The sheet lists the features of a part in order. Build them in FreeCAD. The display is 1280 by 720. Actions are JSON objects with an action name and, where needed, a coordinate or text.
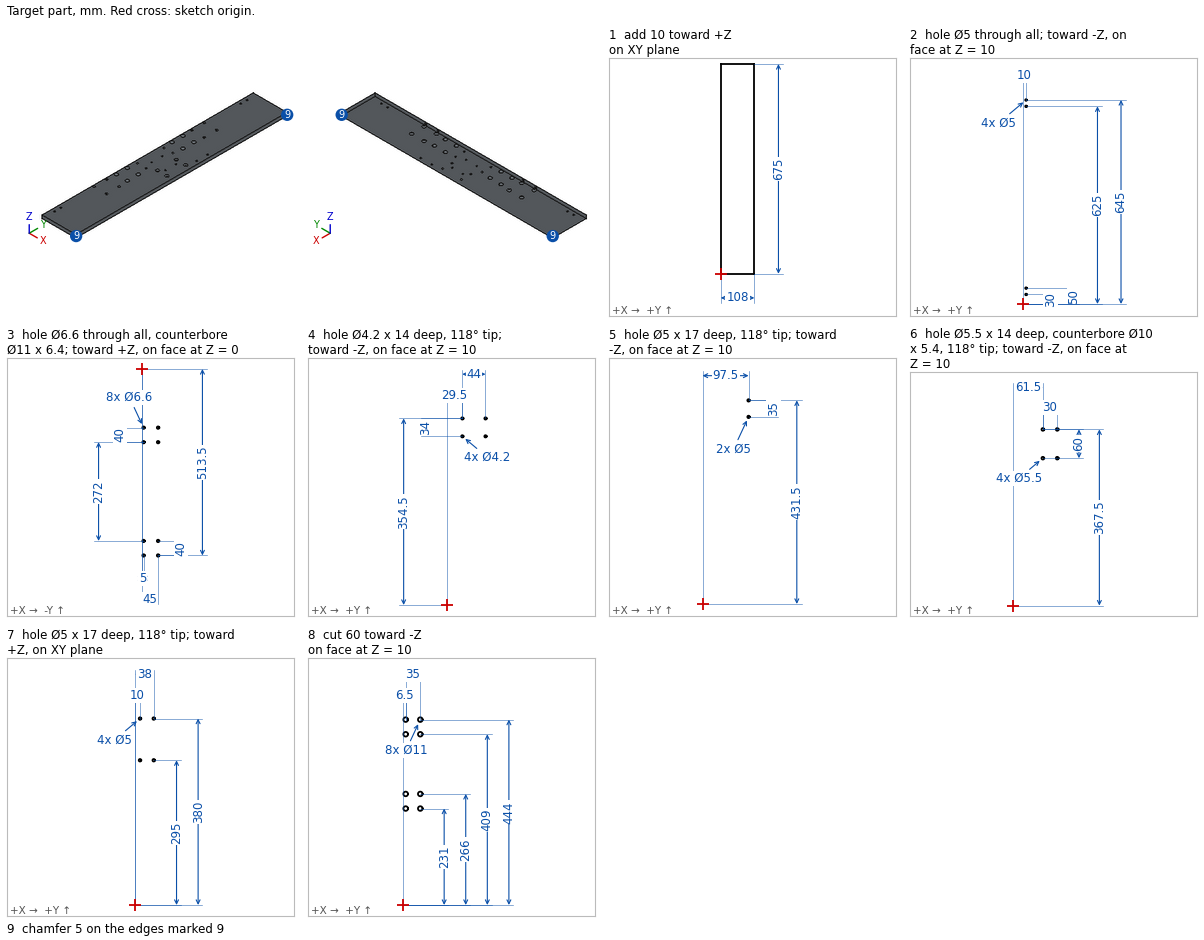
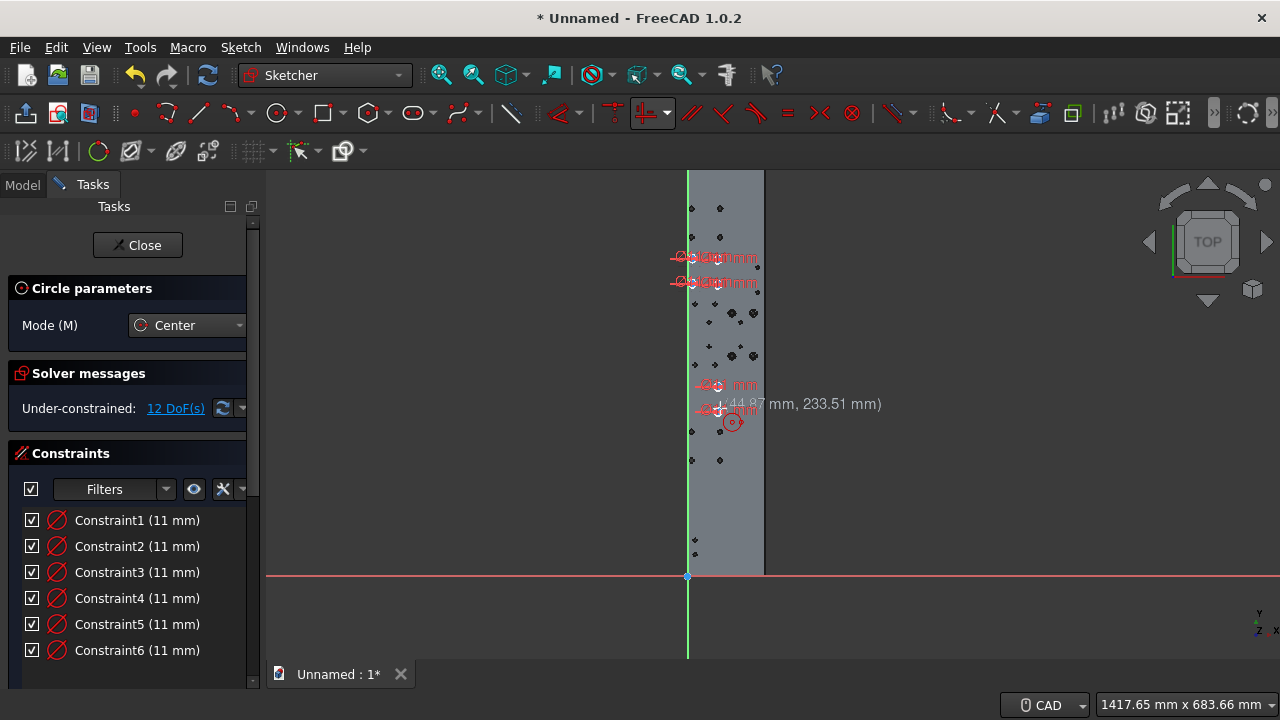
{"action": "scroll", "coordinate": [693, 411], "scroll_direction": "up", "scroll_amount": 9}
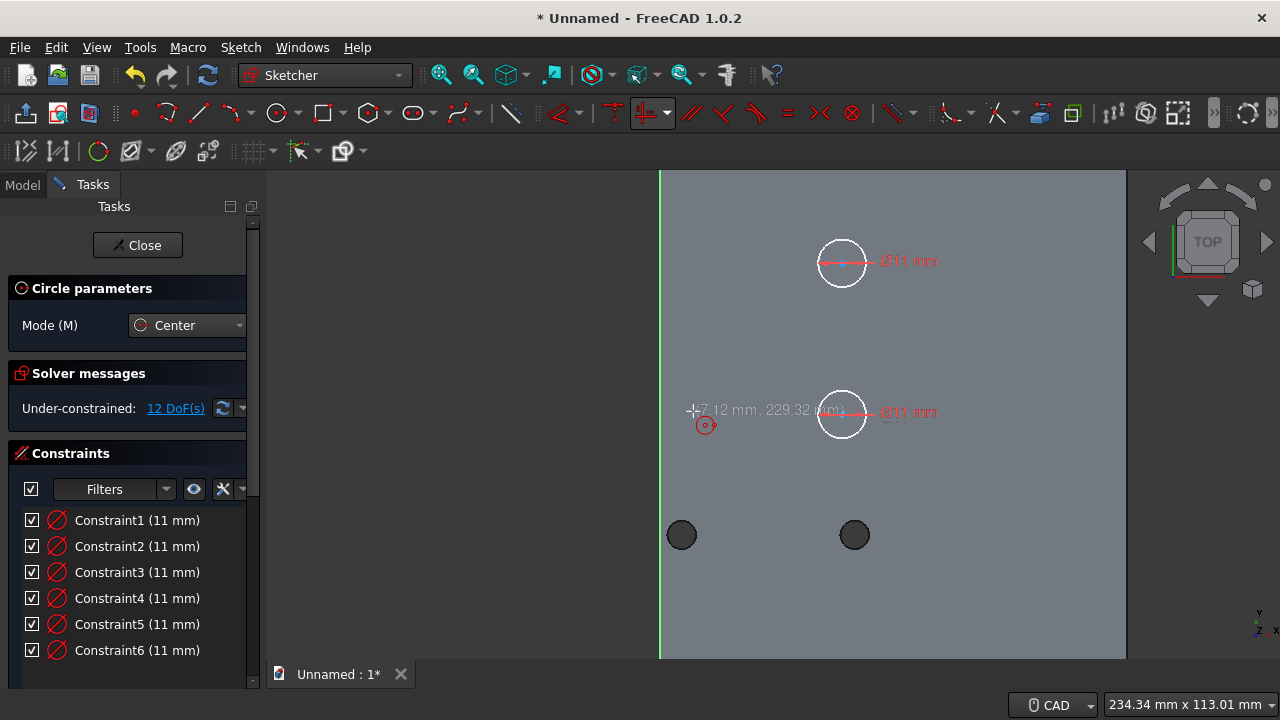
{"action": "left_click", "coordinate": [688, 407]}
{"action": "mouse_move", "coordinate": [705, 390]}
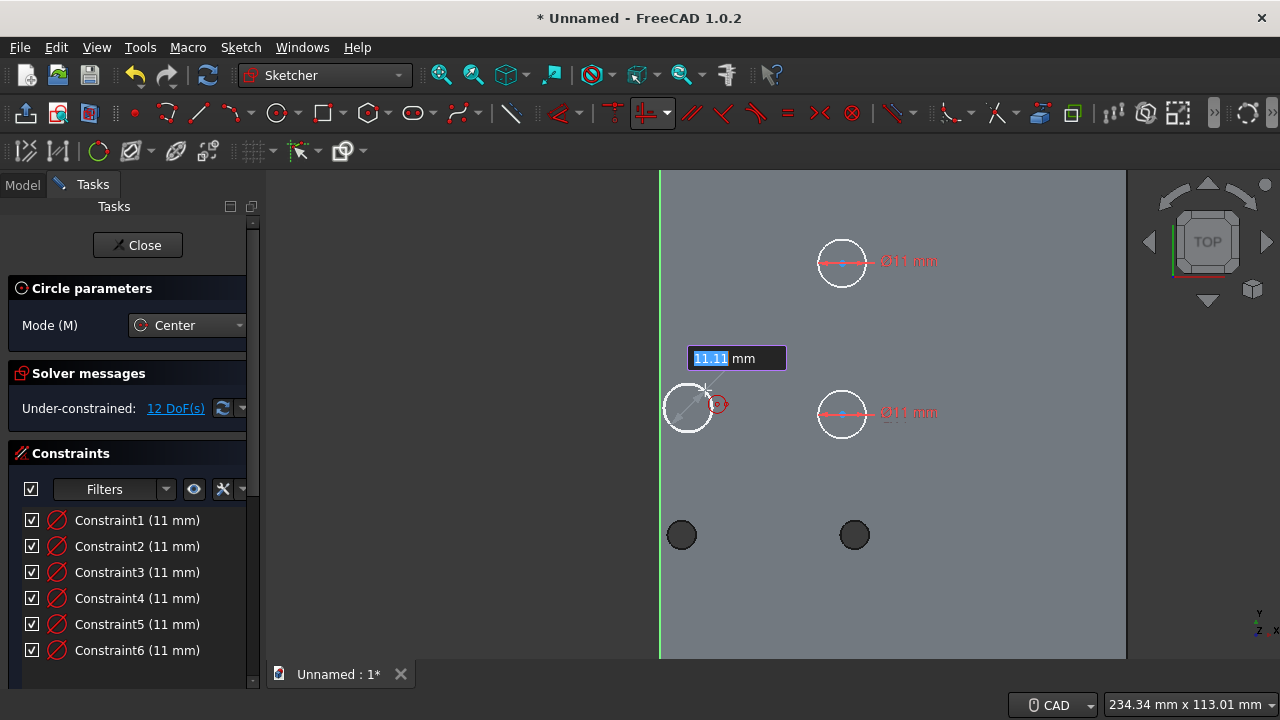
{"action": "type", "text": "11"}
{"action": "key", "text": "Return"}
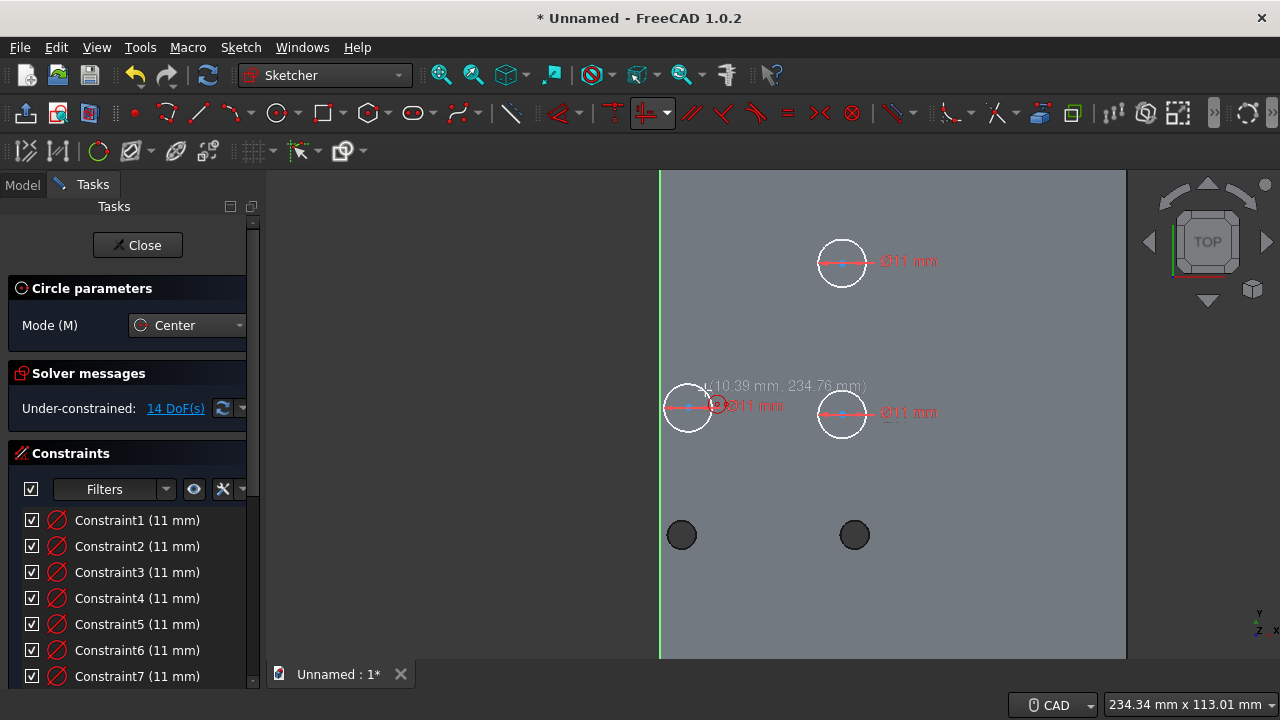
{"action": "left_click", "coordinate": [688, 256]}
{"action": "mouse_move", "coordinate": [705, 239]}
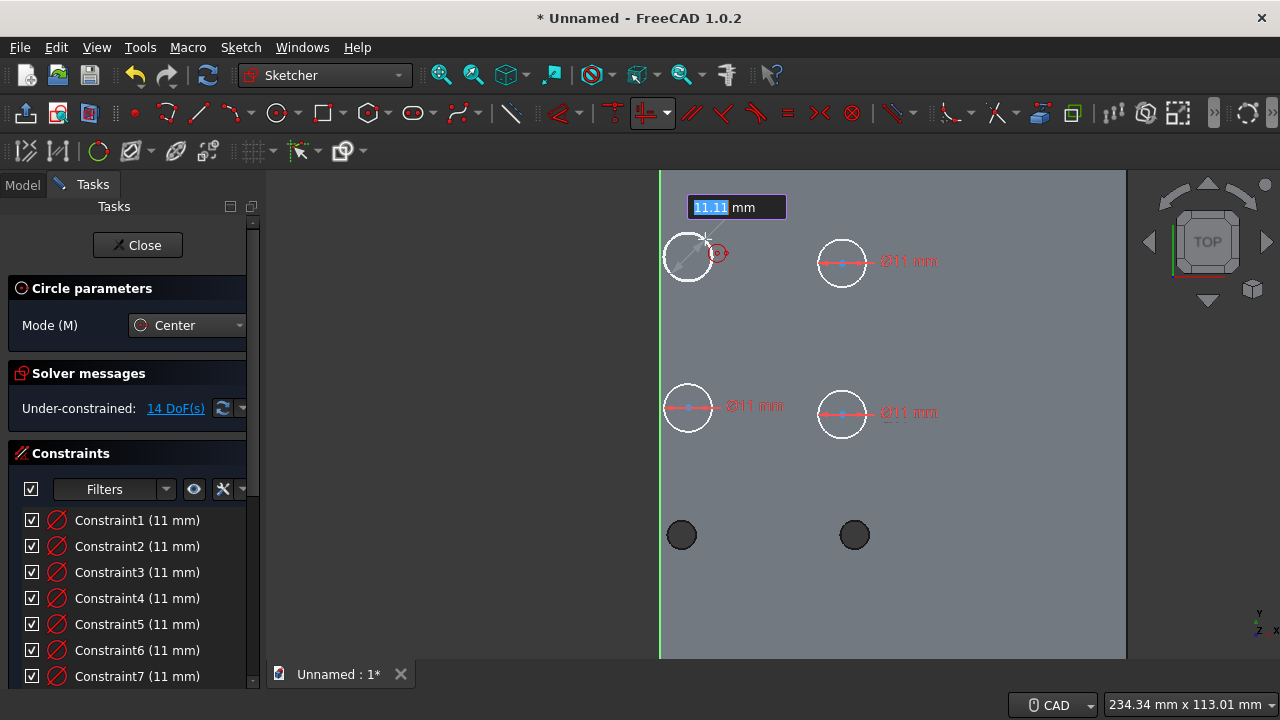
{"action": "type", "text": "11"}
{"action": "key", "text": "Return"}
{"action": "key", "text": "Escape"}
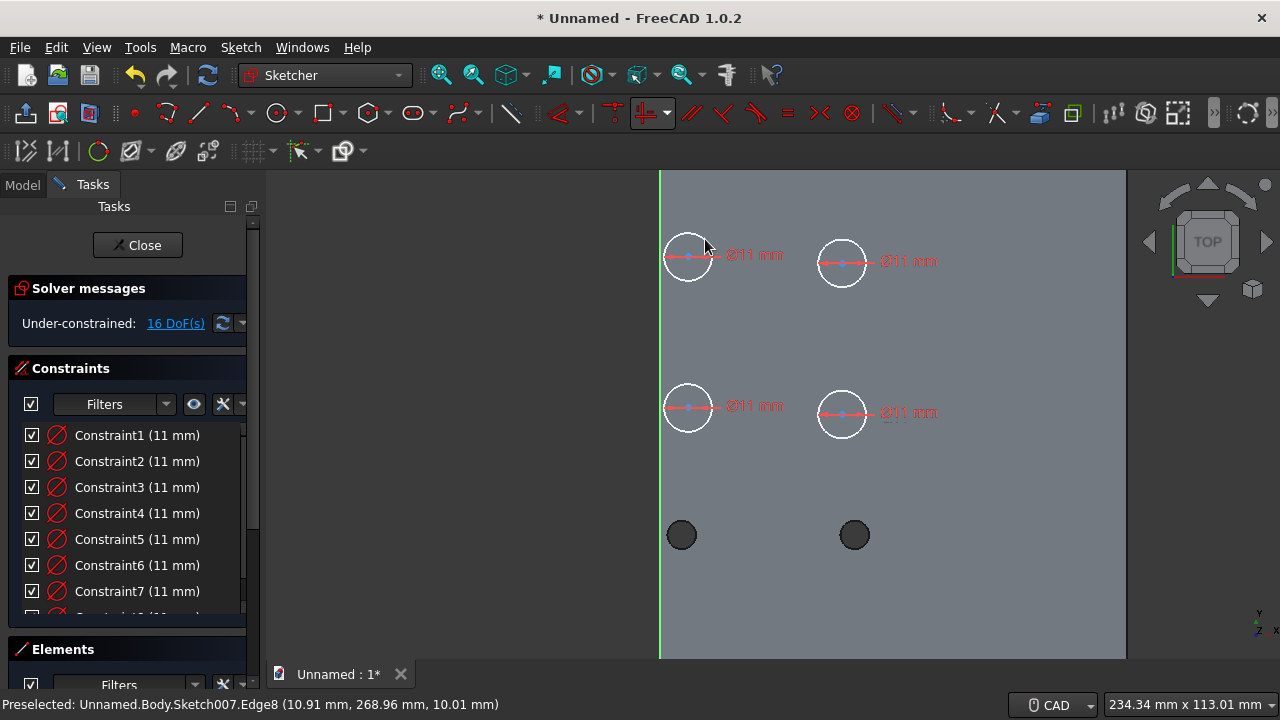
{"action": "scroll", "coordinate": [693, 411], "scroll_direction": "down", "scroll_amount": 9}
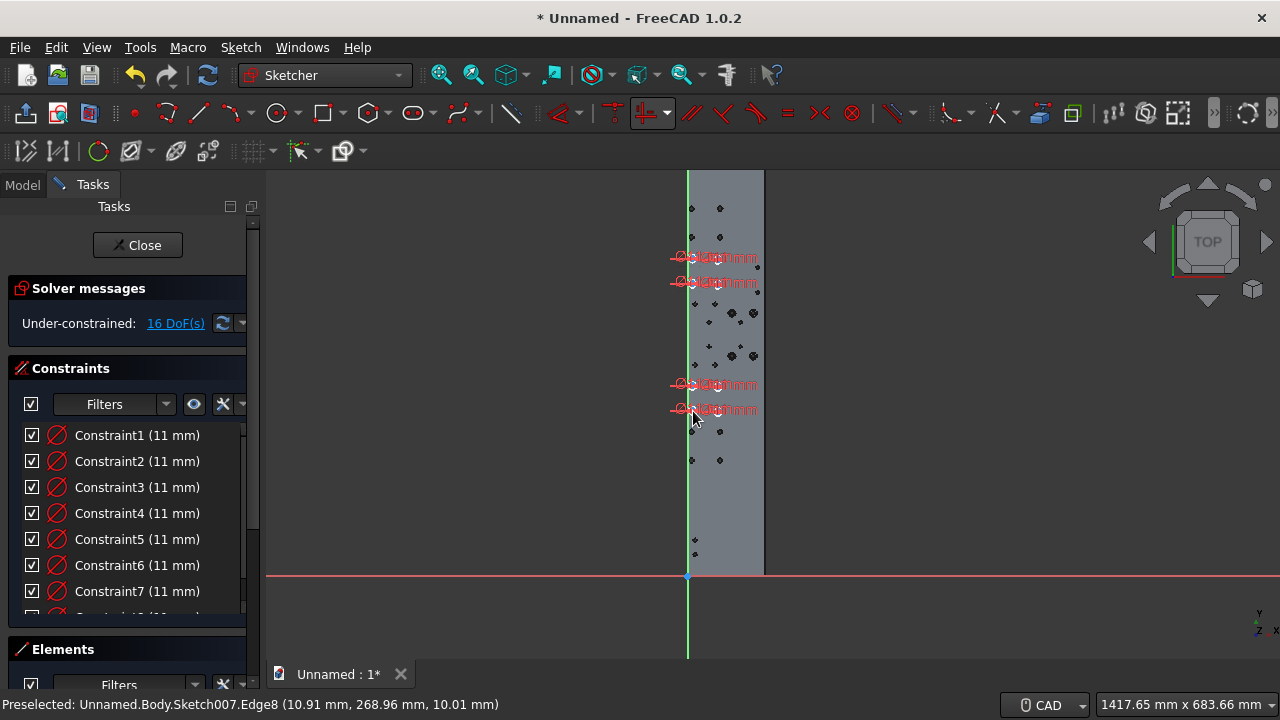
{"action": "left_click", "coordinate": [718, 260]}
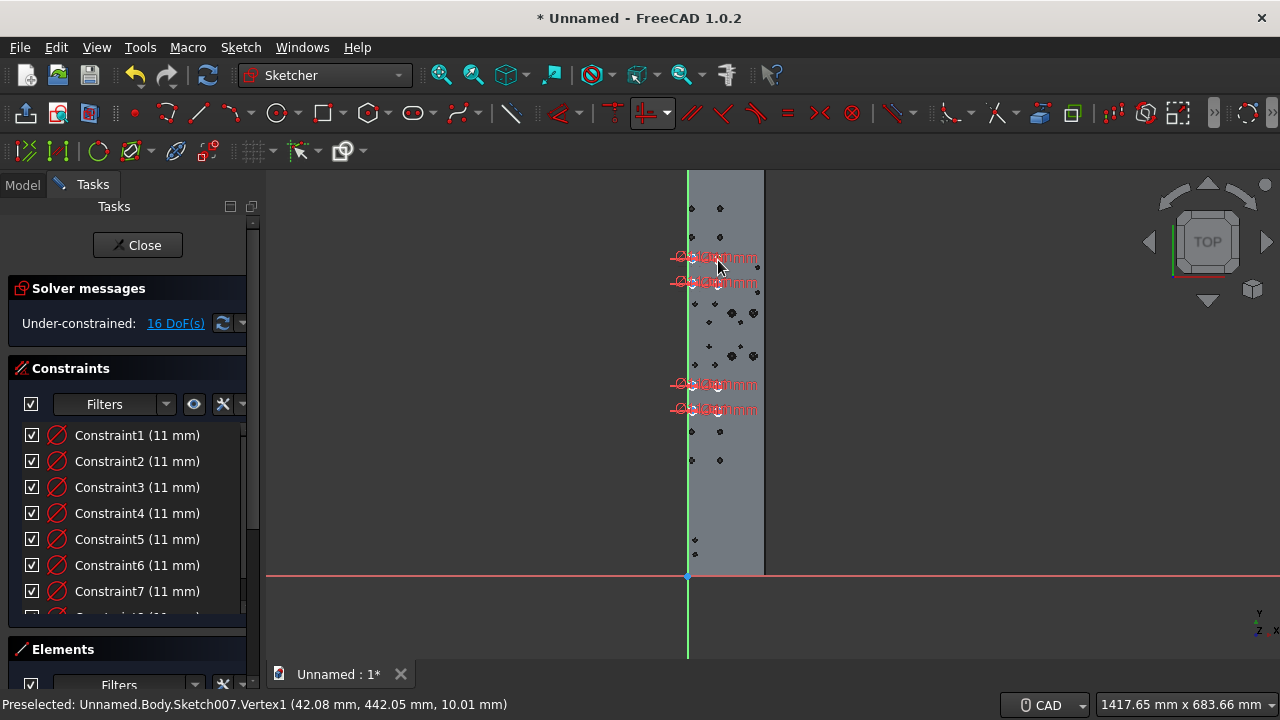
{"action": "left_click", "coordinate": [693, 259]}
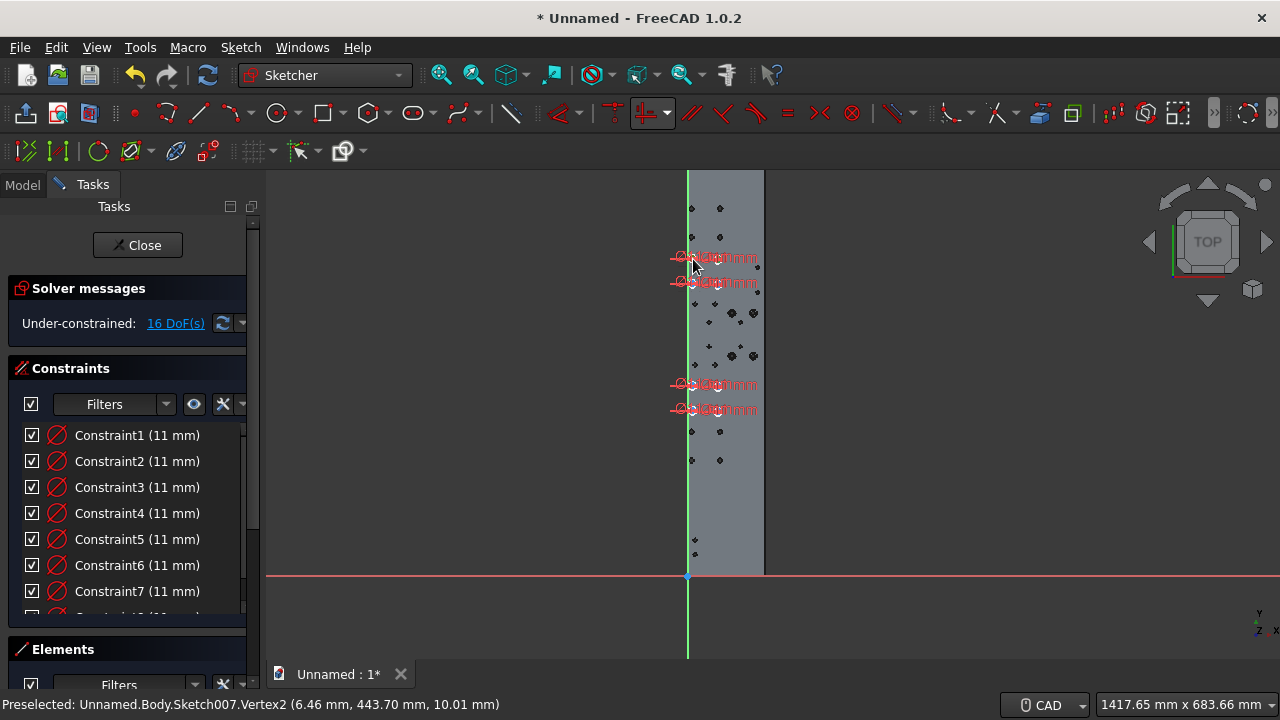
{"action": "left_click", "coordinate": [670, 114]}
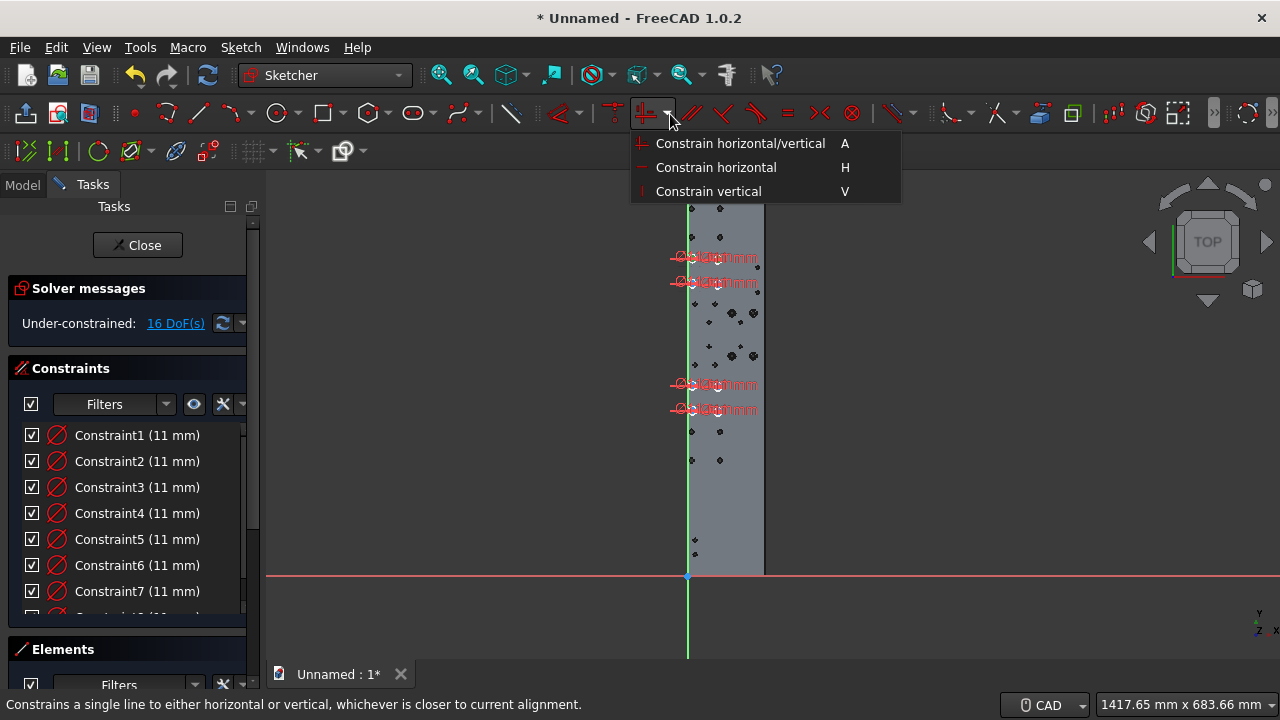
{"action": "left_click", "coordinate": [766, 167]}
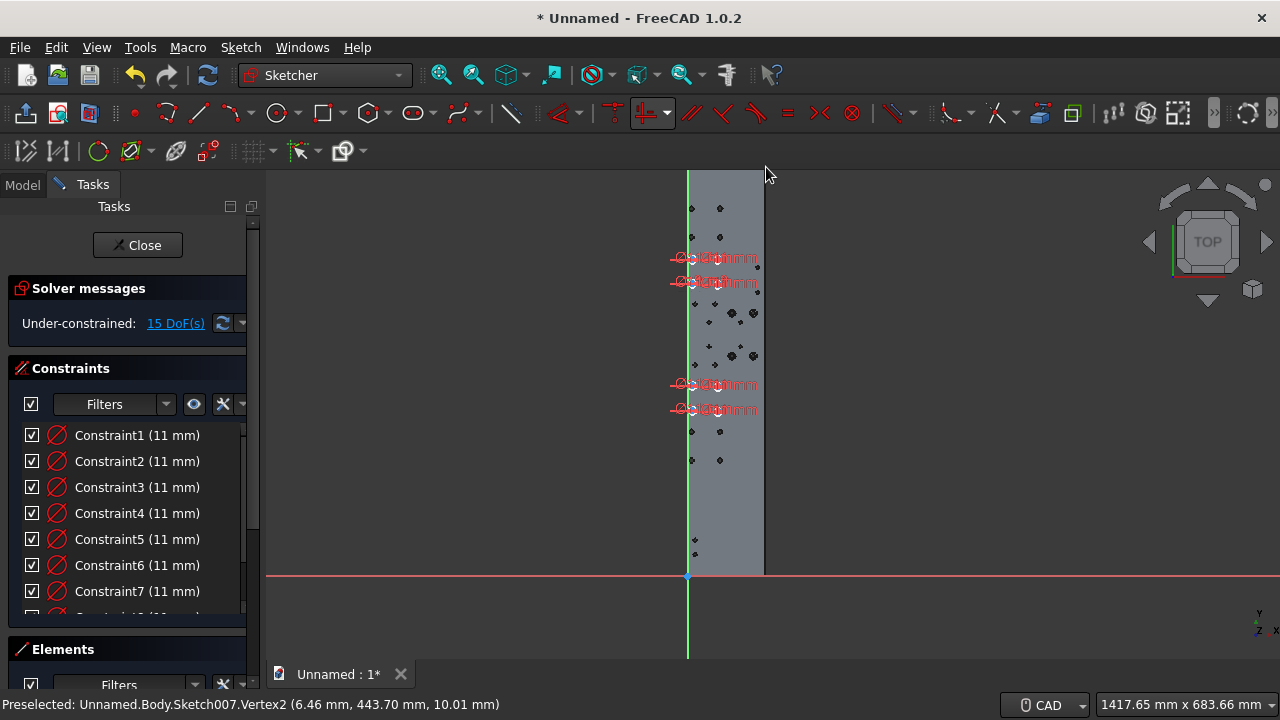
{"action": "left_click", "coordinate": [718, 260]}